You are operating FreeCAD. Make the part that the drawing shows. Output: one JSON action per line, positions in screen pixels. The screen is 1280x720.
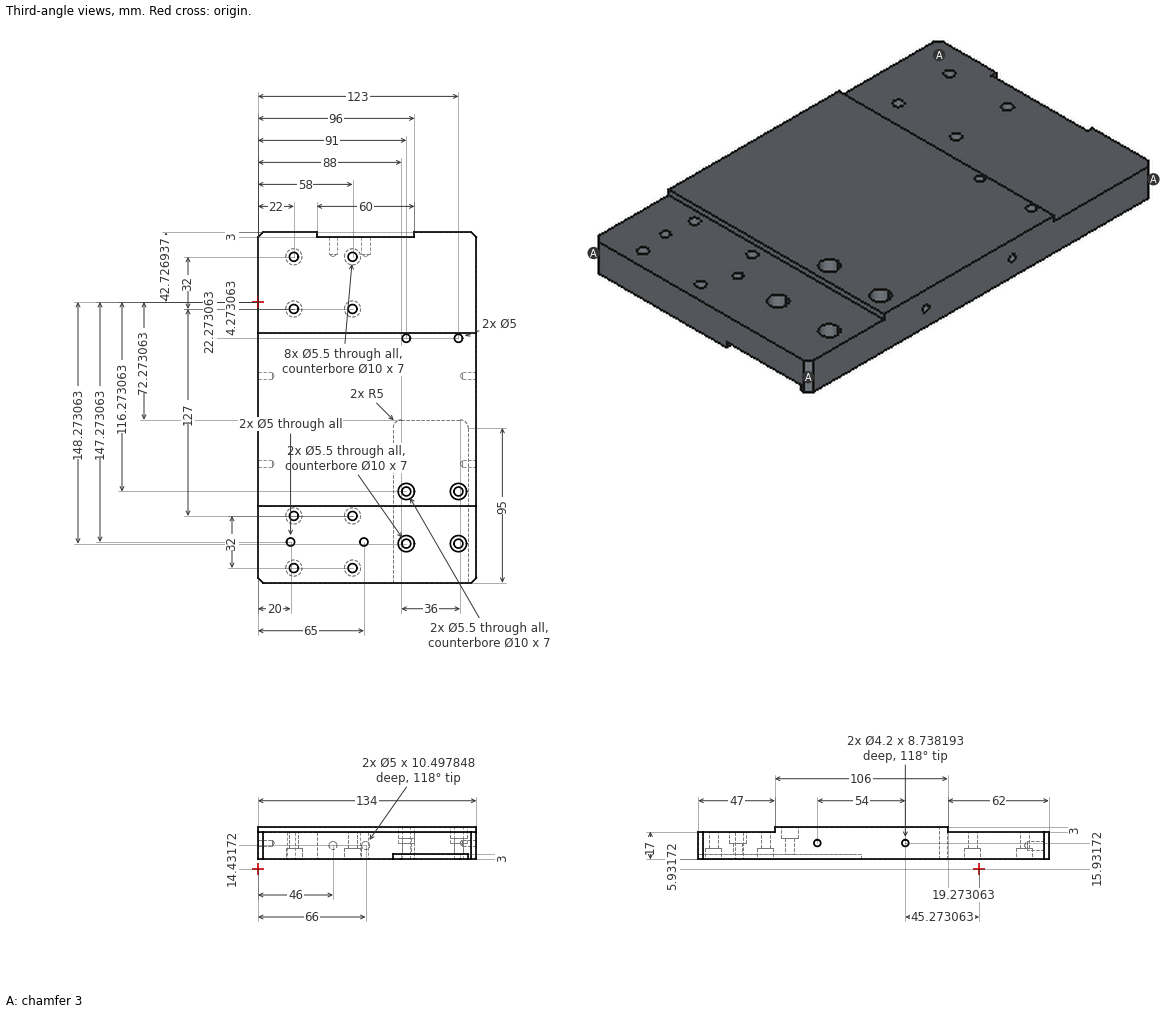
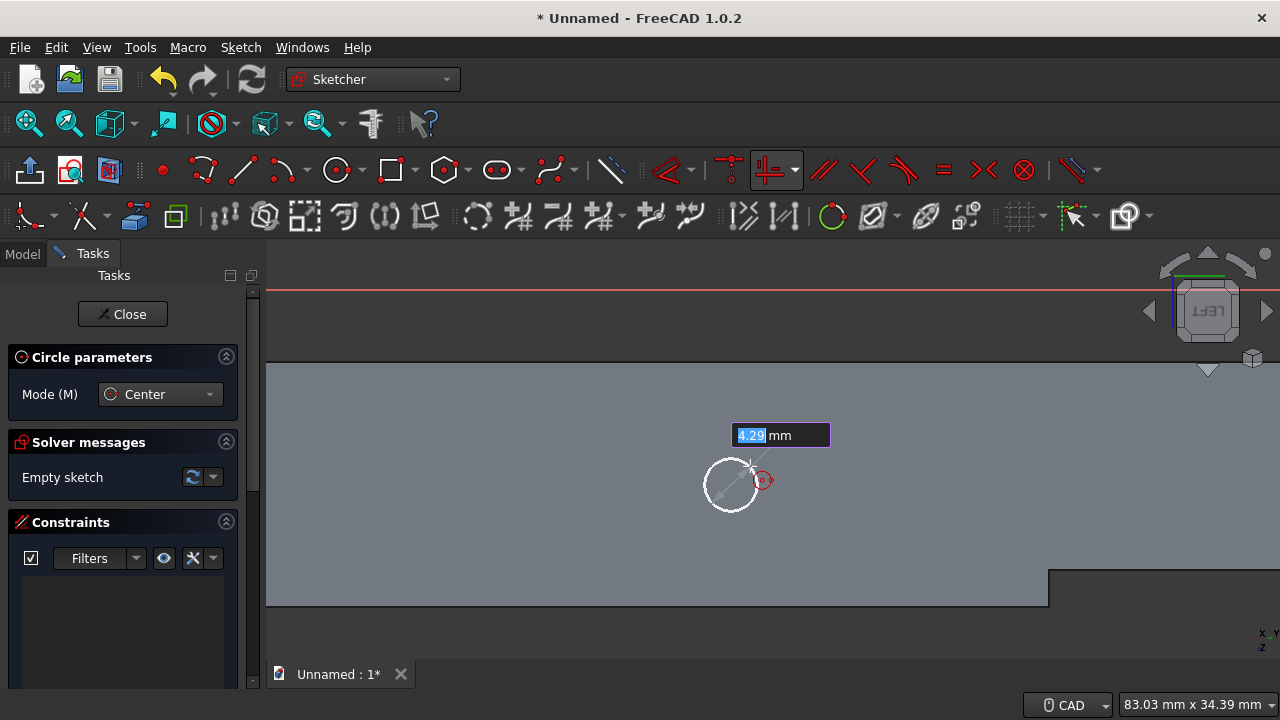
{"action": "type", "text": "4.2"}
{"action": "key", "text": "Return"}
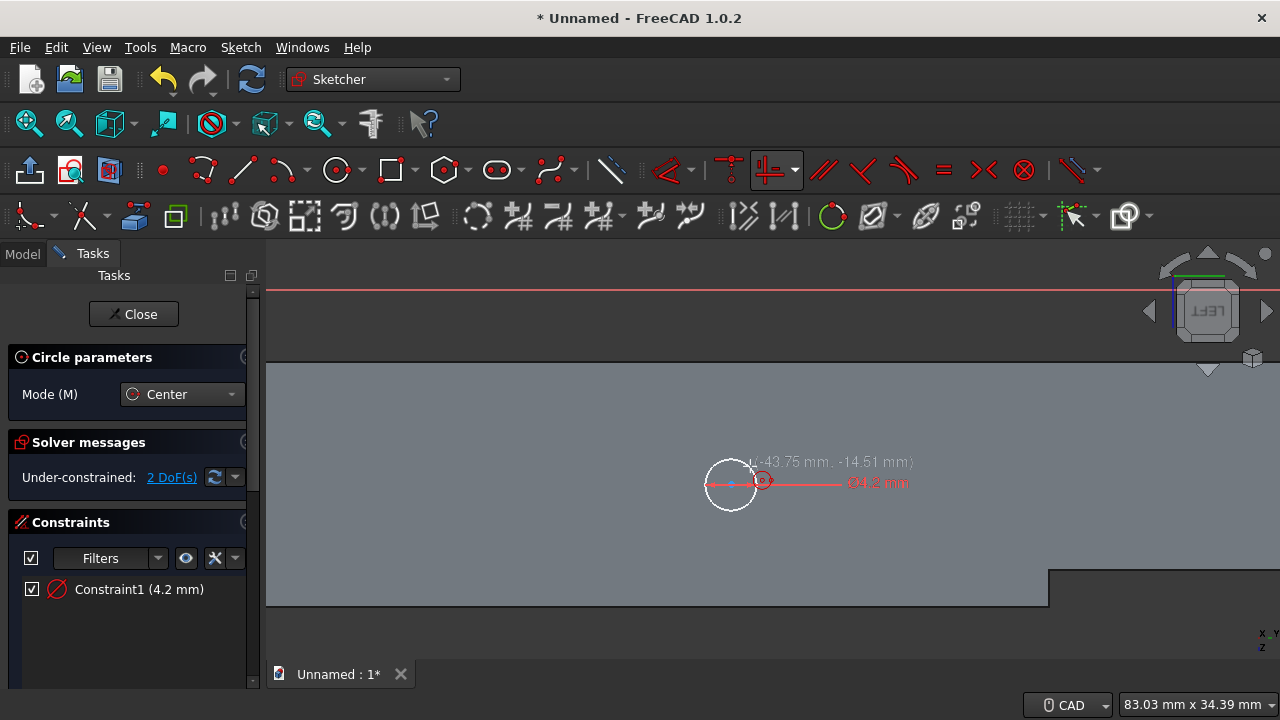
{"action": "scroll", "coordinate": [737, 489], "scroll_direction": "down", "scroll_amount": 4}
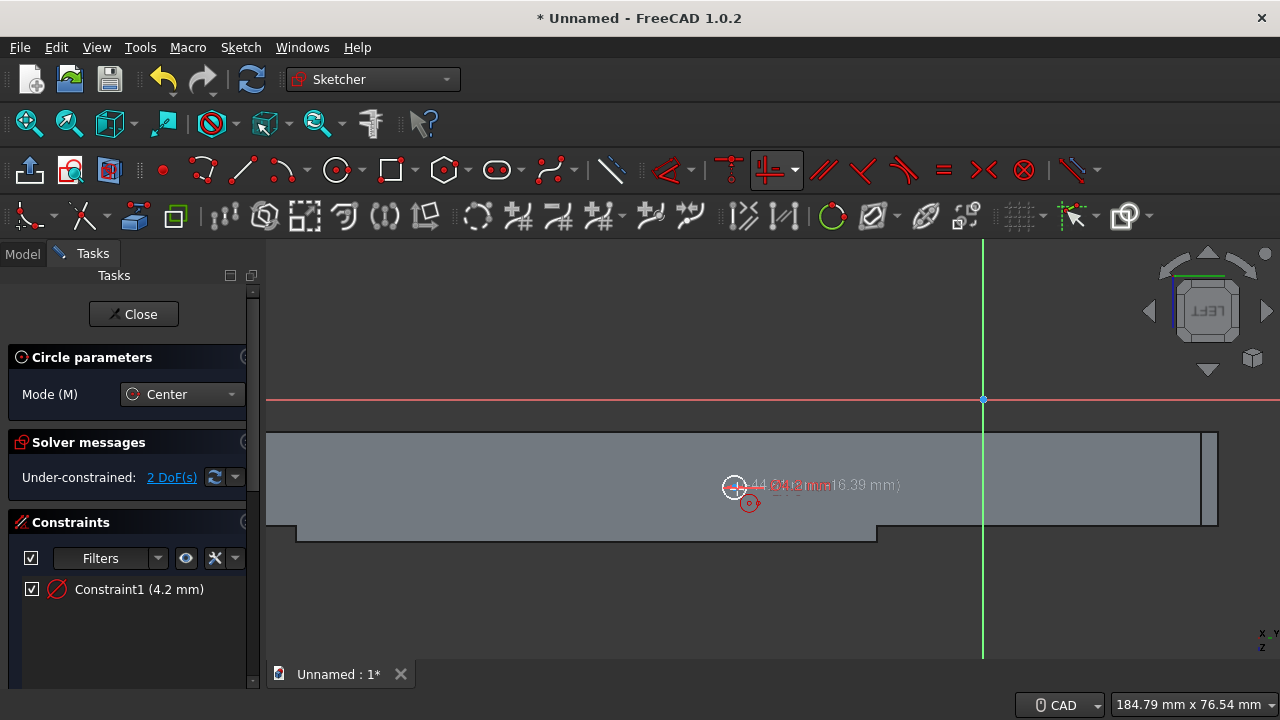
{"action": "scroll", "coordinate": [438, 487], "scroll_direction": "up", "scroll_amount": 4}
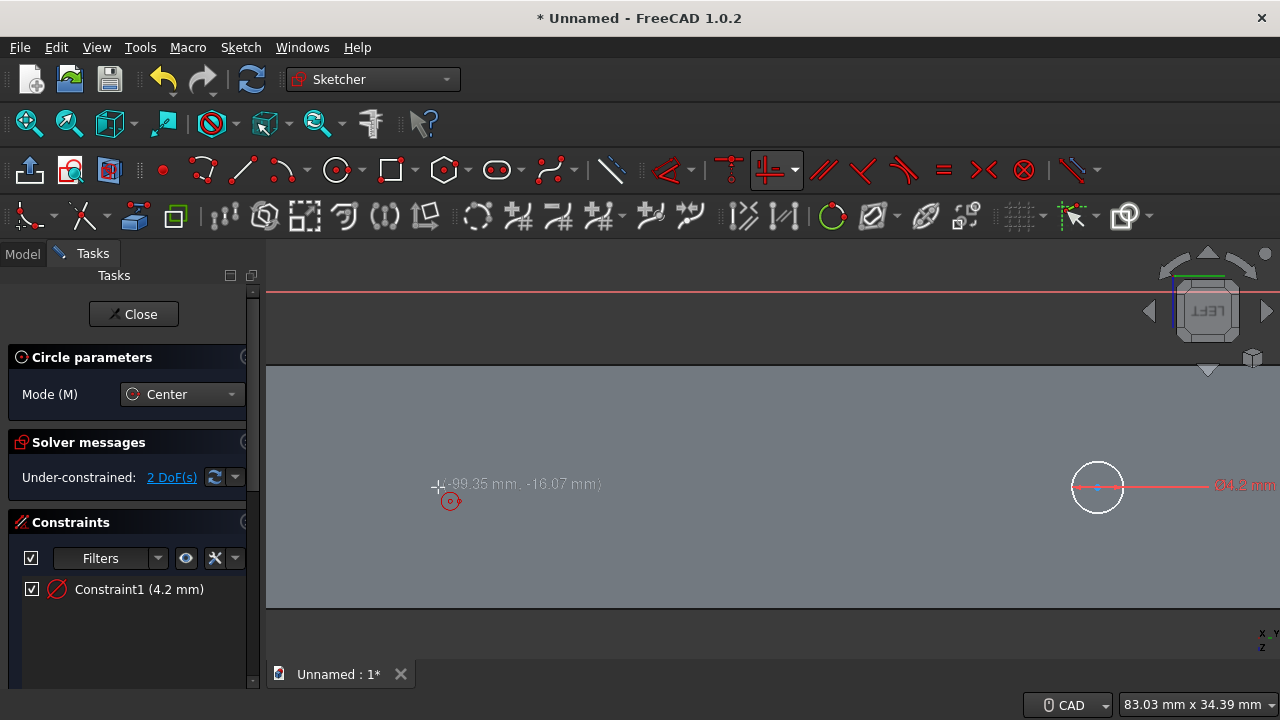
{"action": "left_click", "coordinate": [439, 487]}
{"action": "mouse_move", "coordinate": [457, 469]}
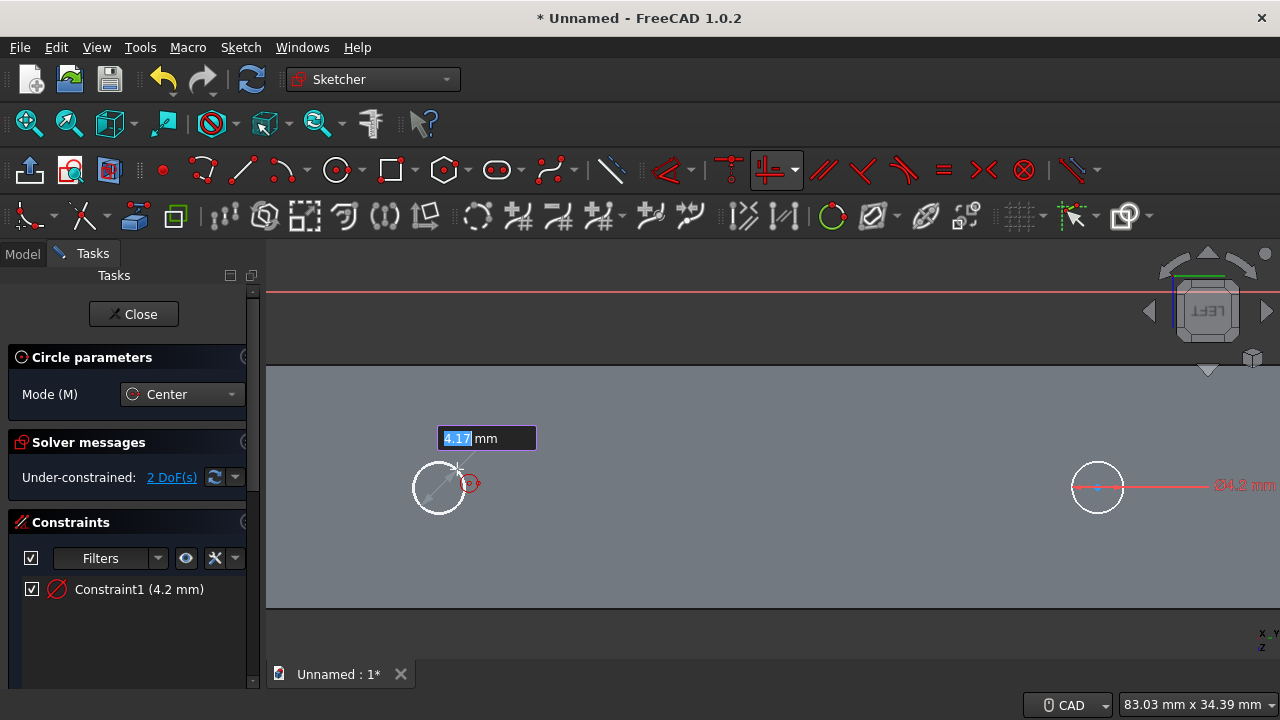
{"action": "type", "text": "4.2"}
{"action": "key", "text": "Return"}
{"action": "key", "text": "Escape"}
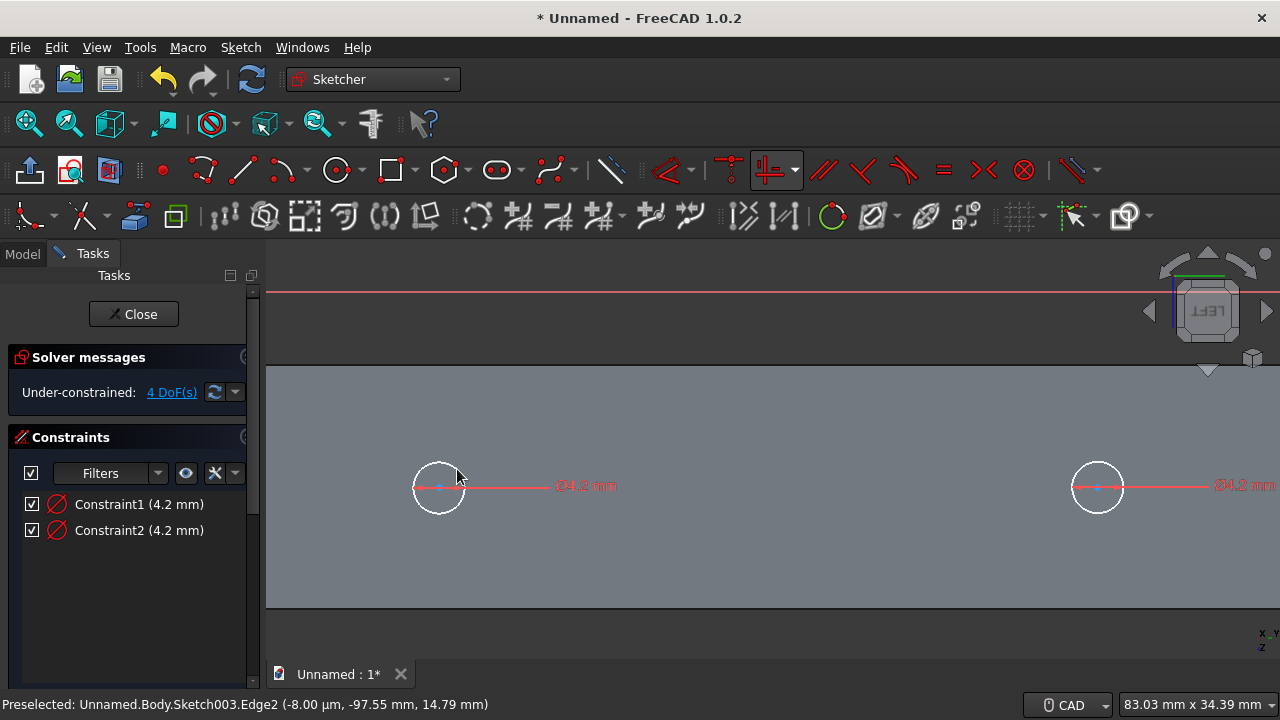
{"action": "left_click", "coordinate": [1098, 487]}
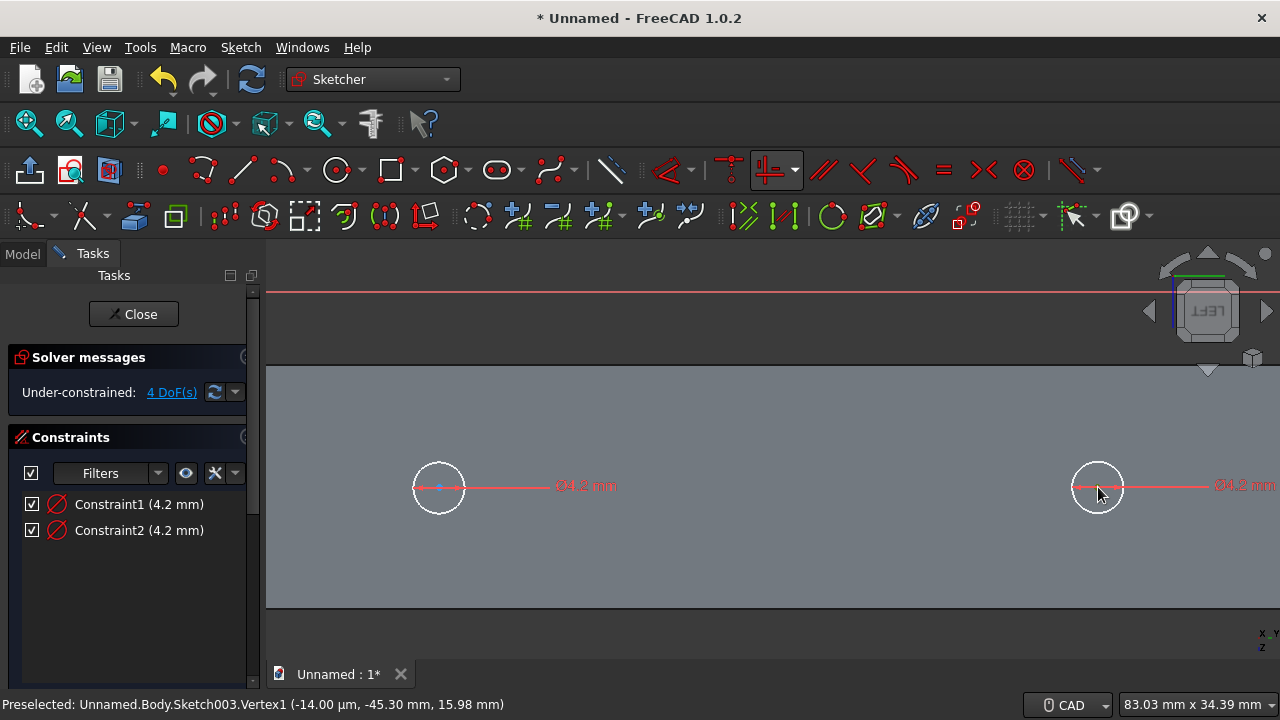
{"action": "left_click", "coordinate": [439, 488]}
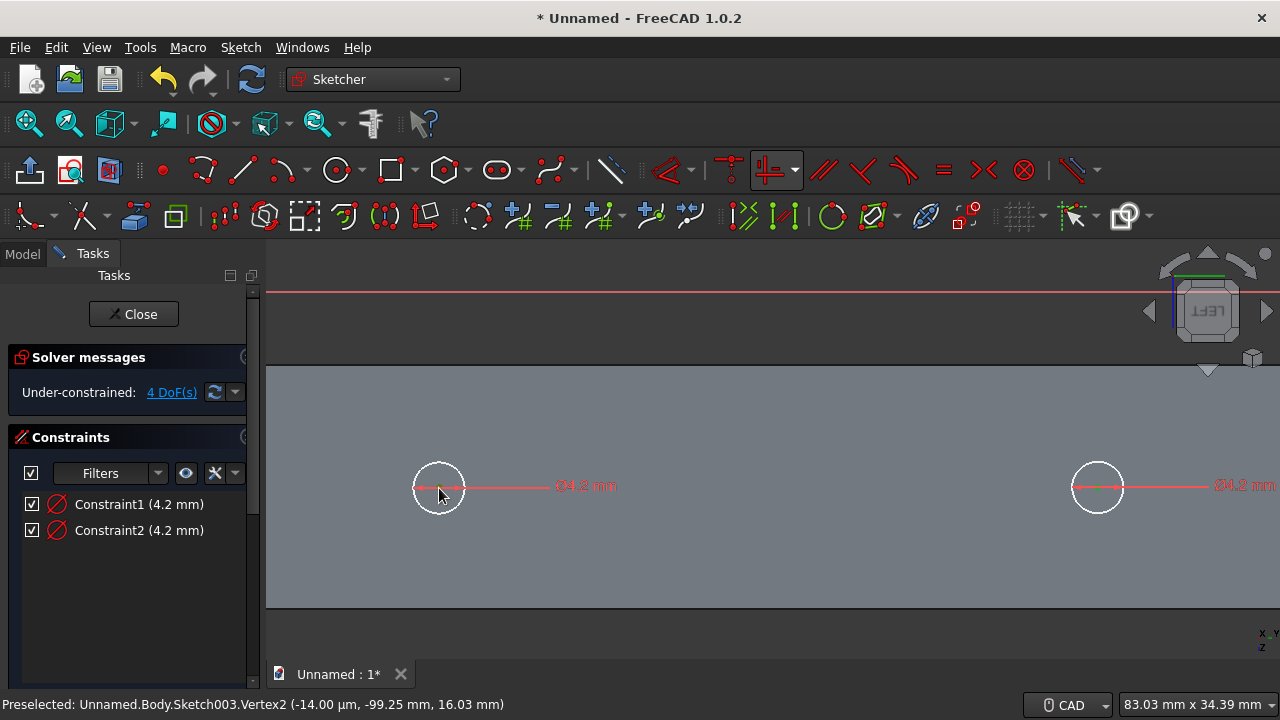
{"action": "left_click", "coordinate": [798, 170]}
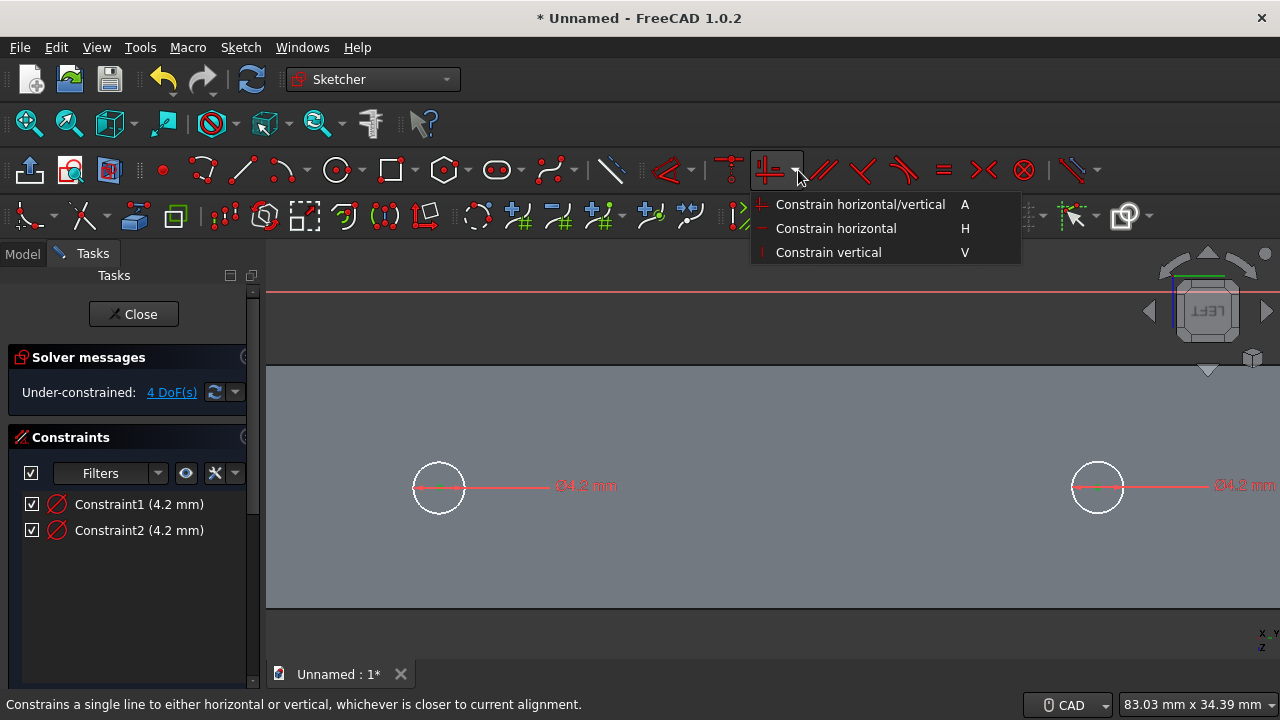
{"action": "left_click", "coordinate": [886, 228]}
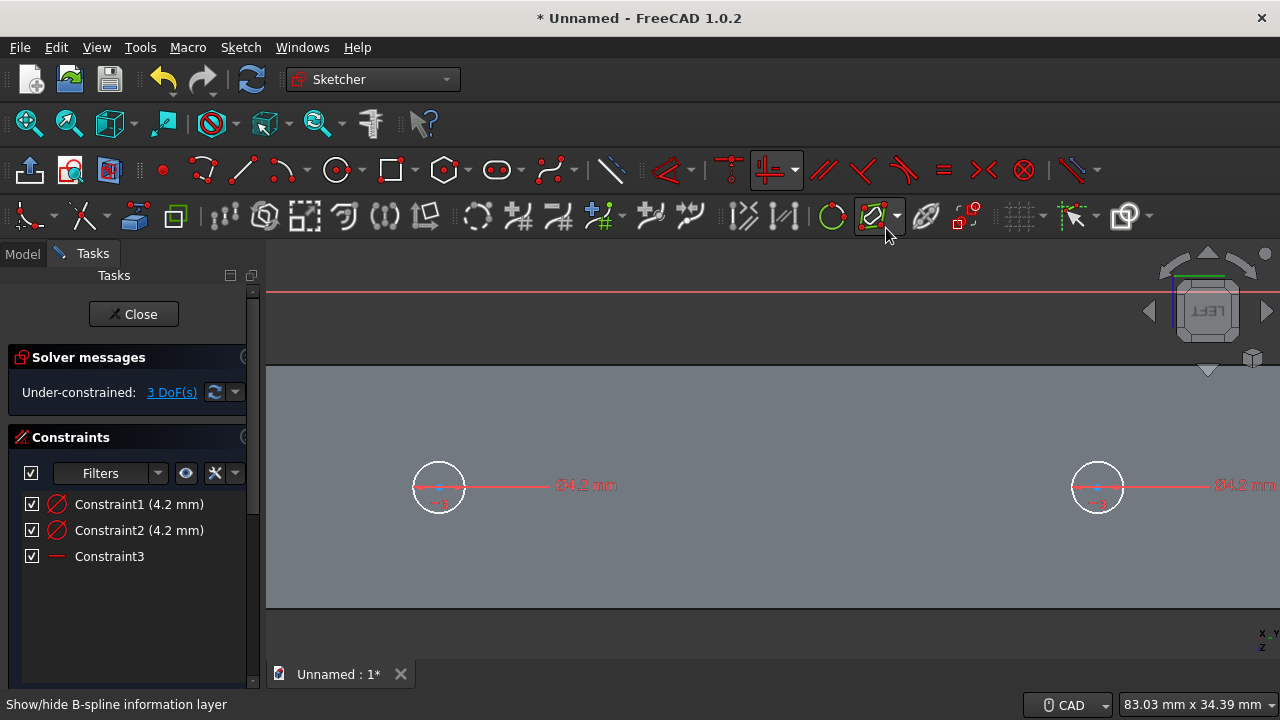
{"action": "left_click", "coordinate": [666, 170]}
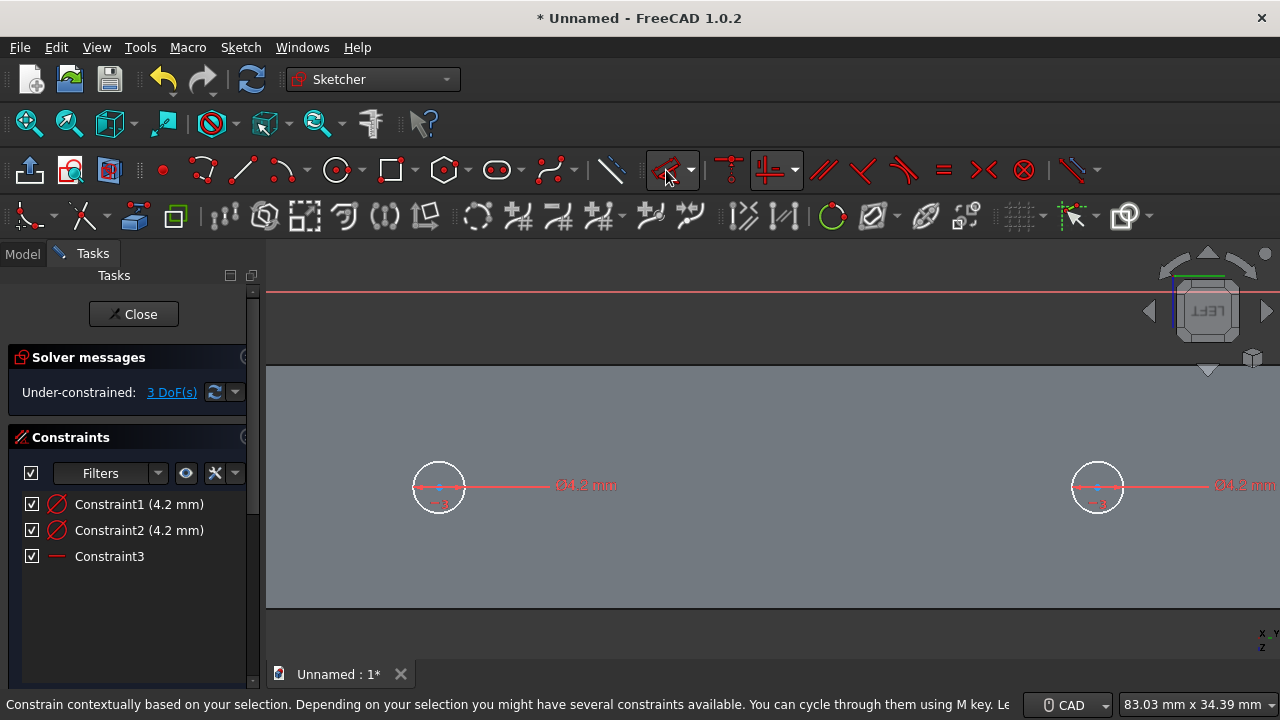
{"action": "left_click", "coordinate": [1098, 487]}